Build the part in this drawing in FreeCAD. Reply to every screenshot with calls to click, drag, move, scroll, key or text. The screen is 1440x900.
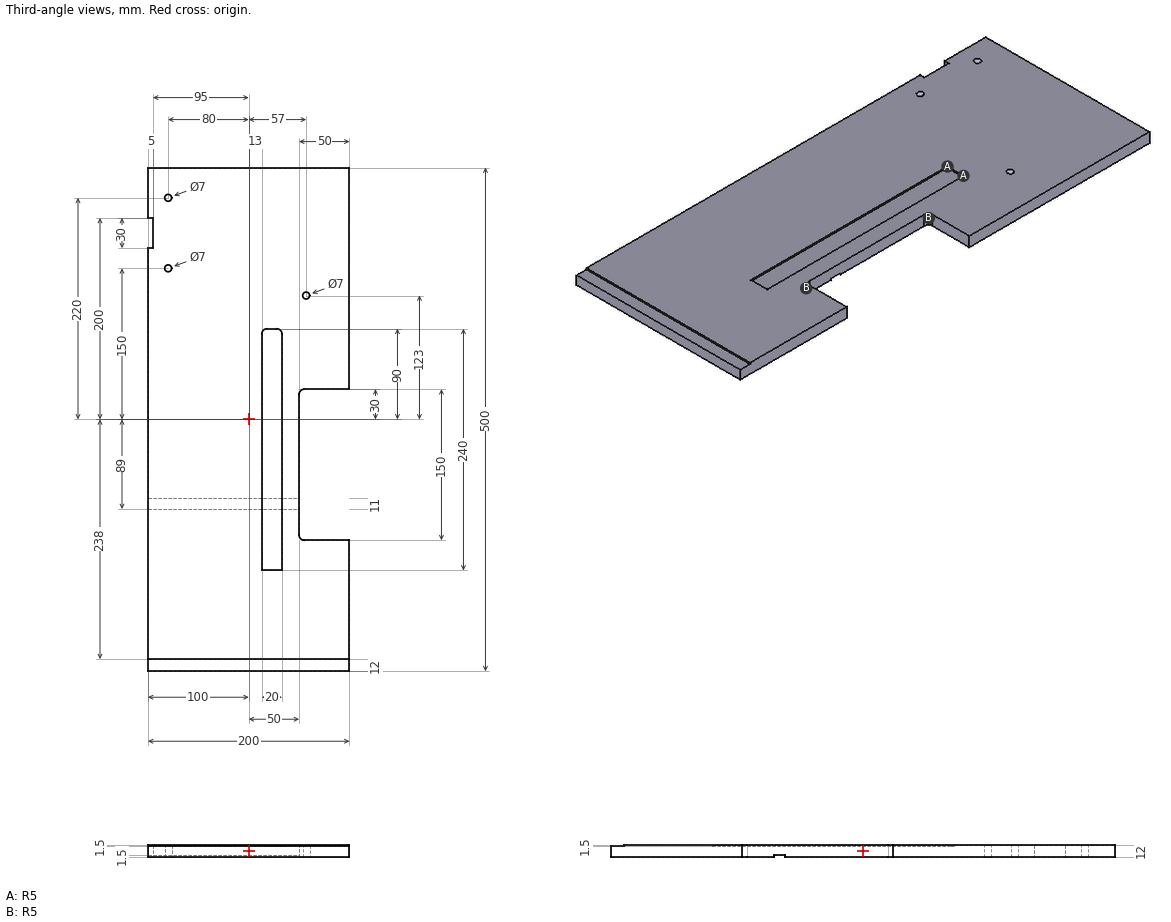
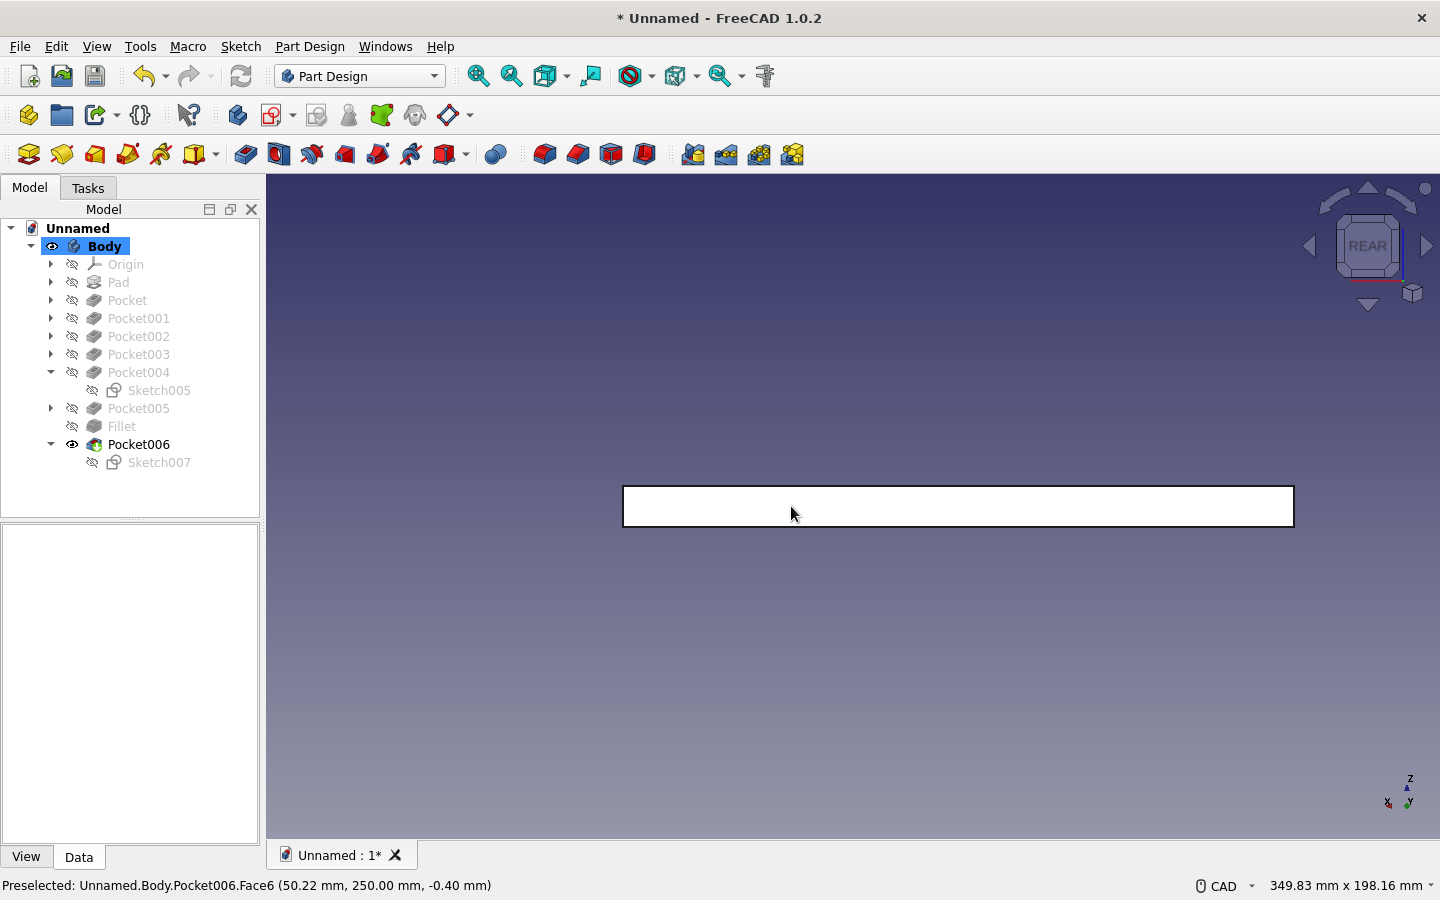
click(479, 76)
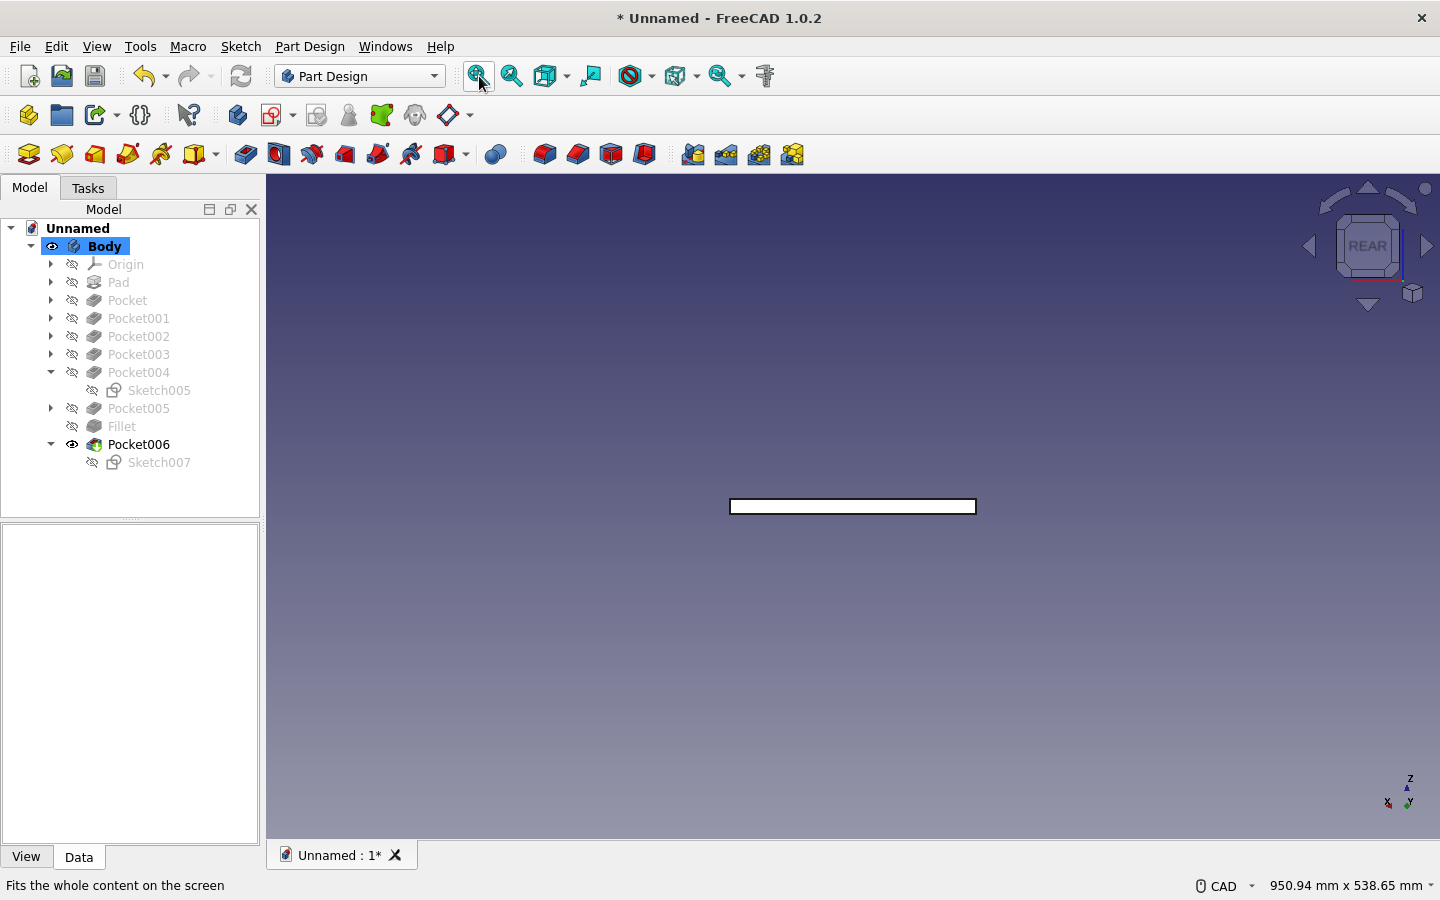
key(6)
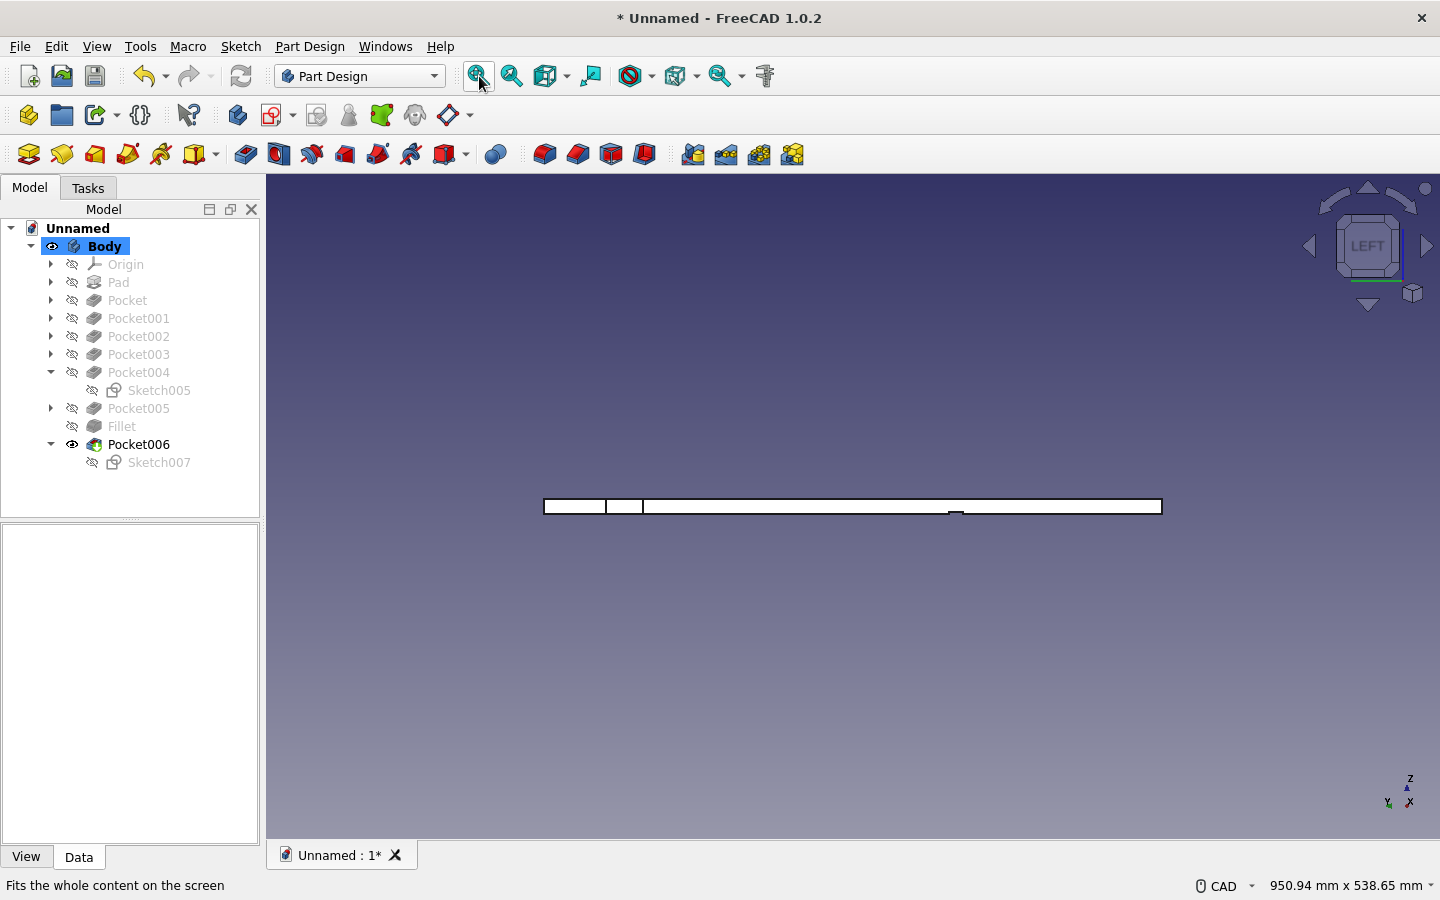
scroll(816, 505, up, 5)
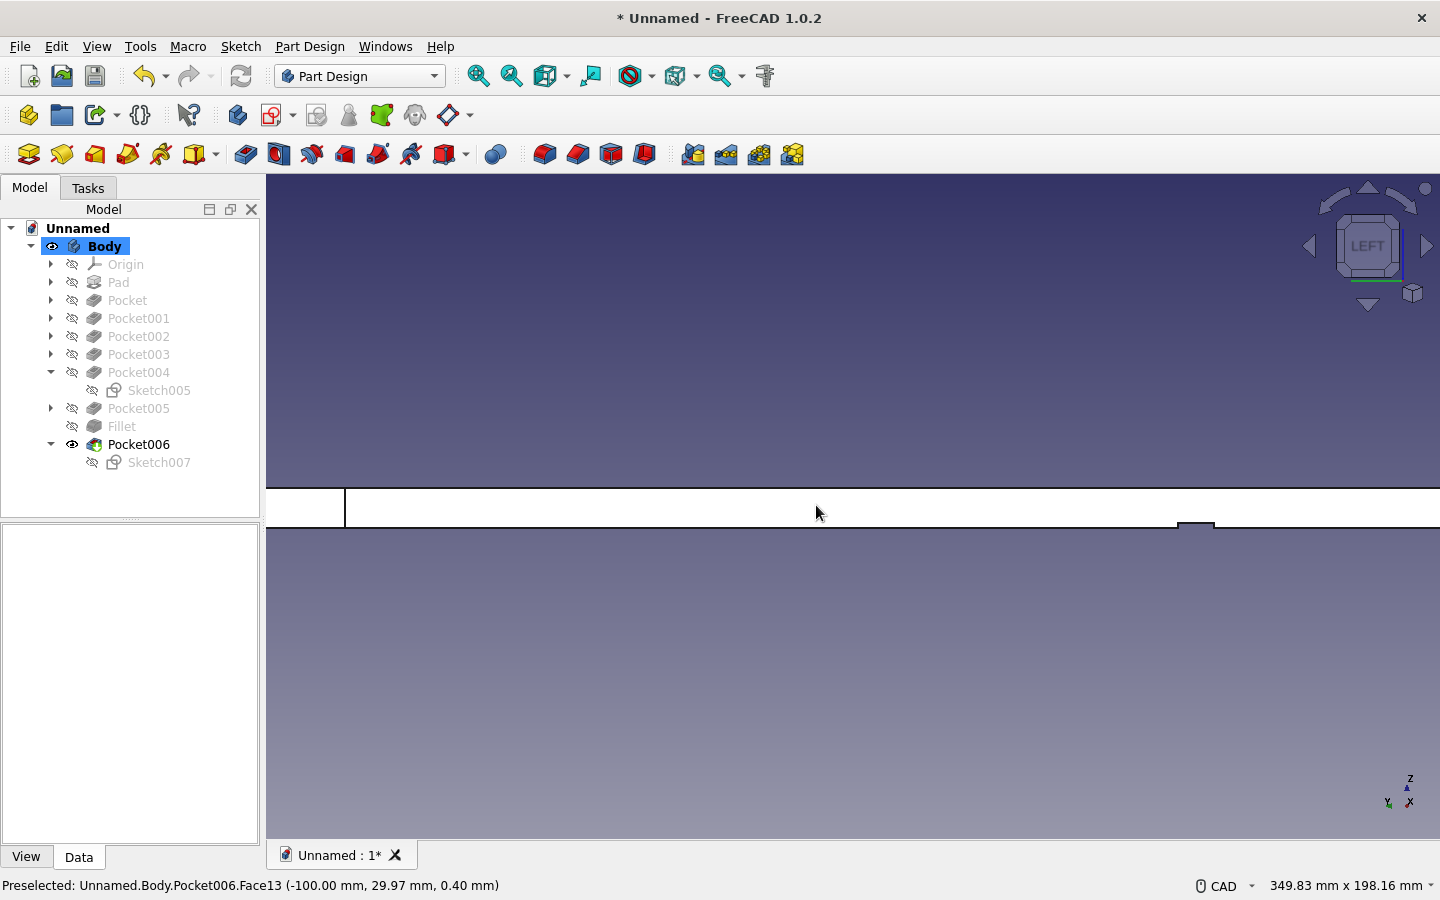
click(479, 76)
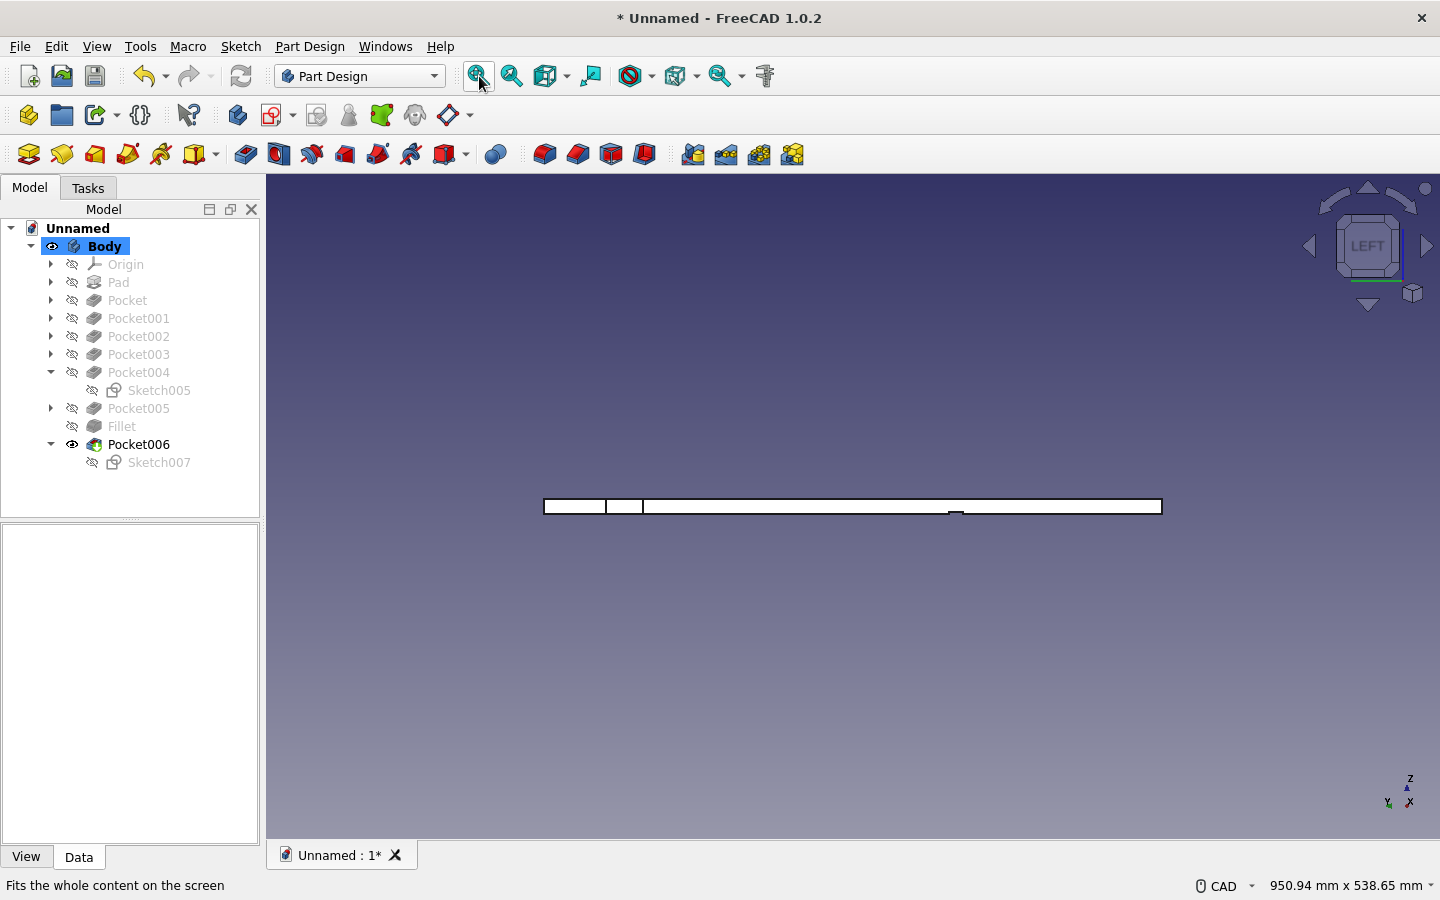
key(v)
key(3)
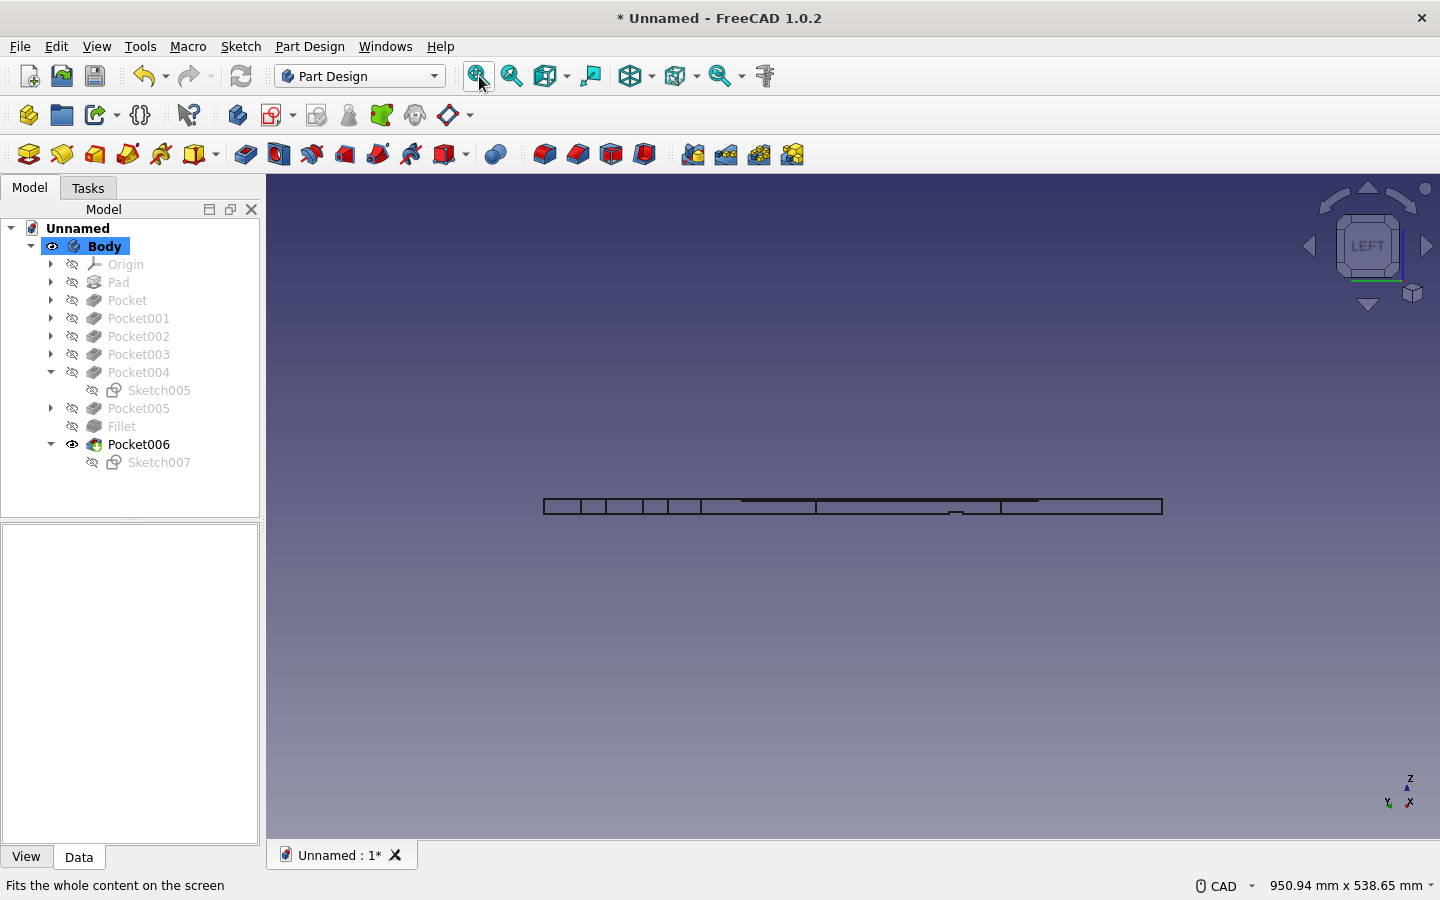
key(0)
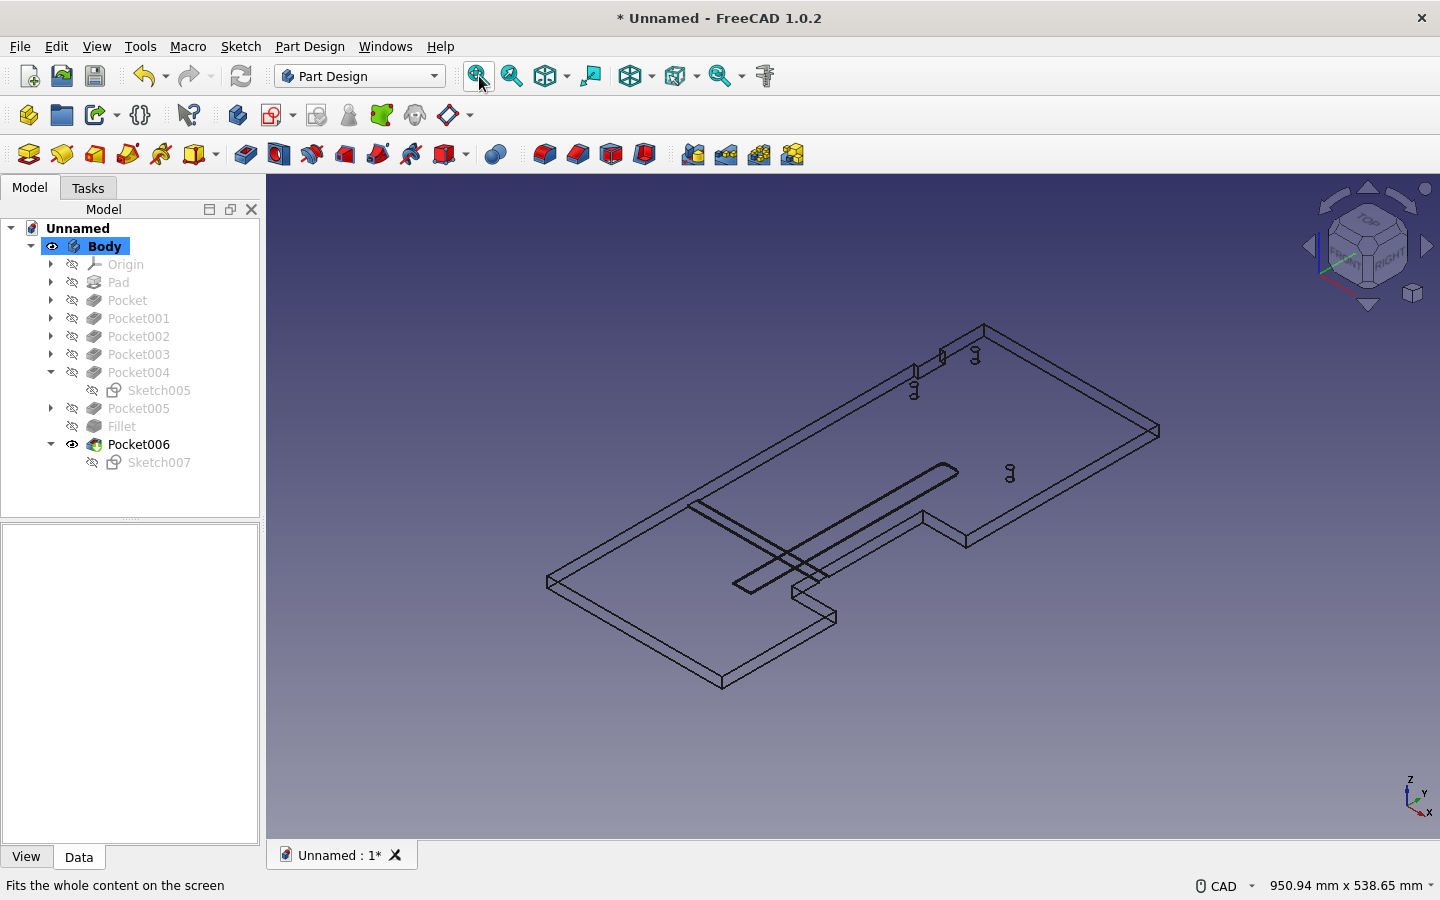
click(923, 517)